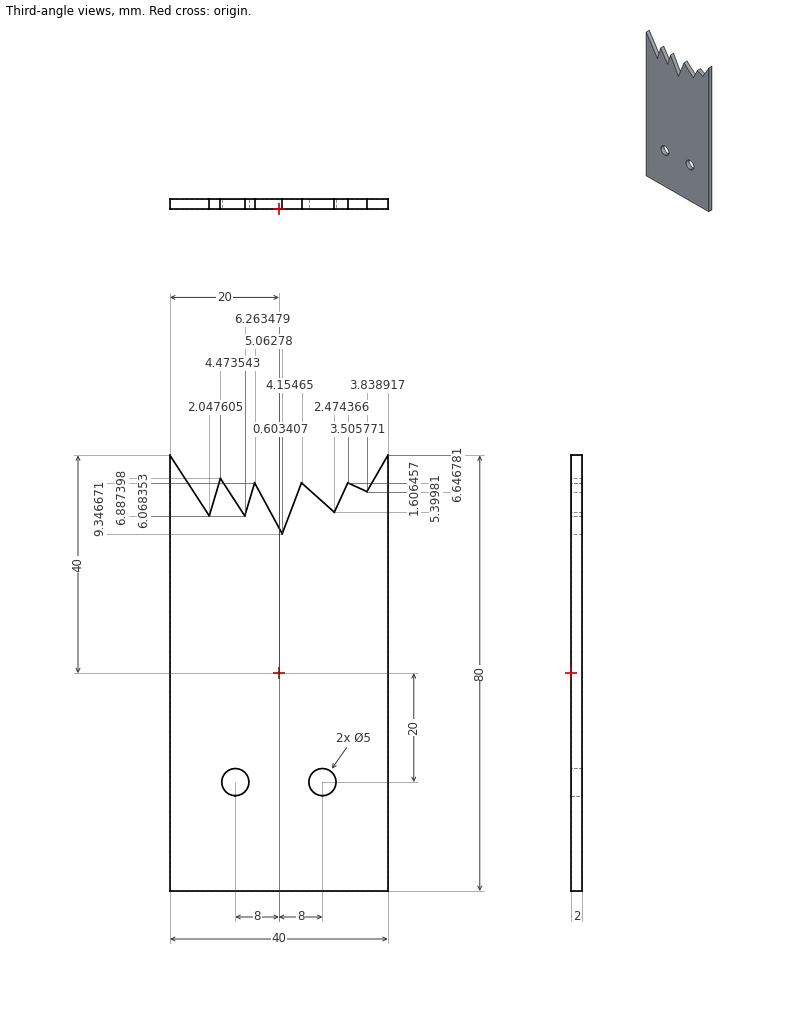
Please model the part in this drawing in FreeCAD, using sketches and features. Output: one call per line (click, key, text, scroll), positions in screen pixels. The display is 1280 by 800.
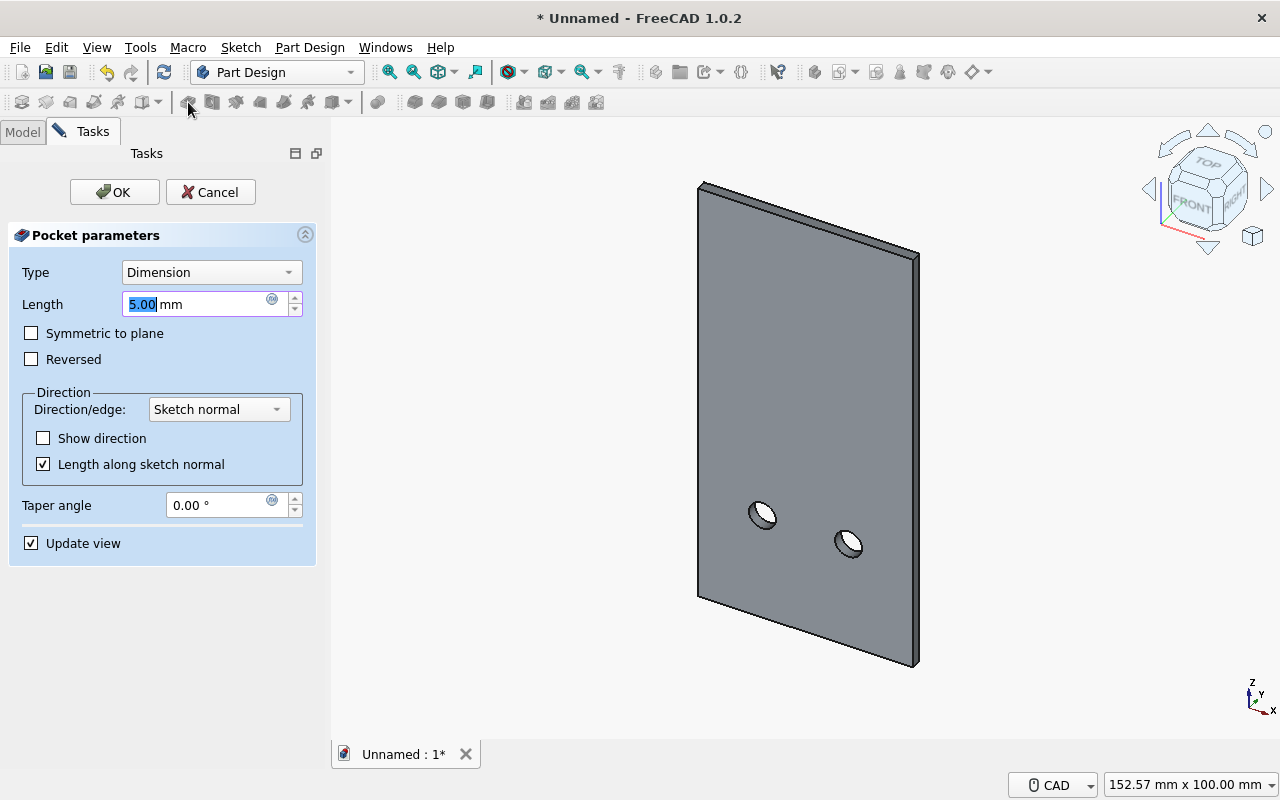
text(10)
key(Tab)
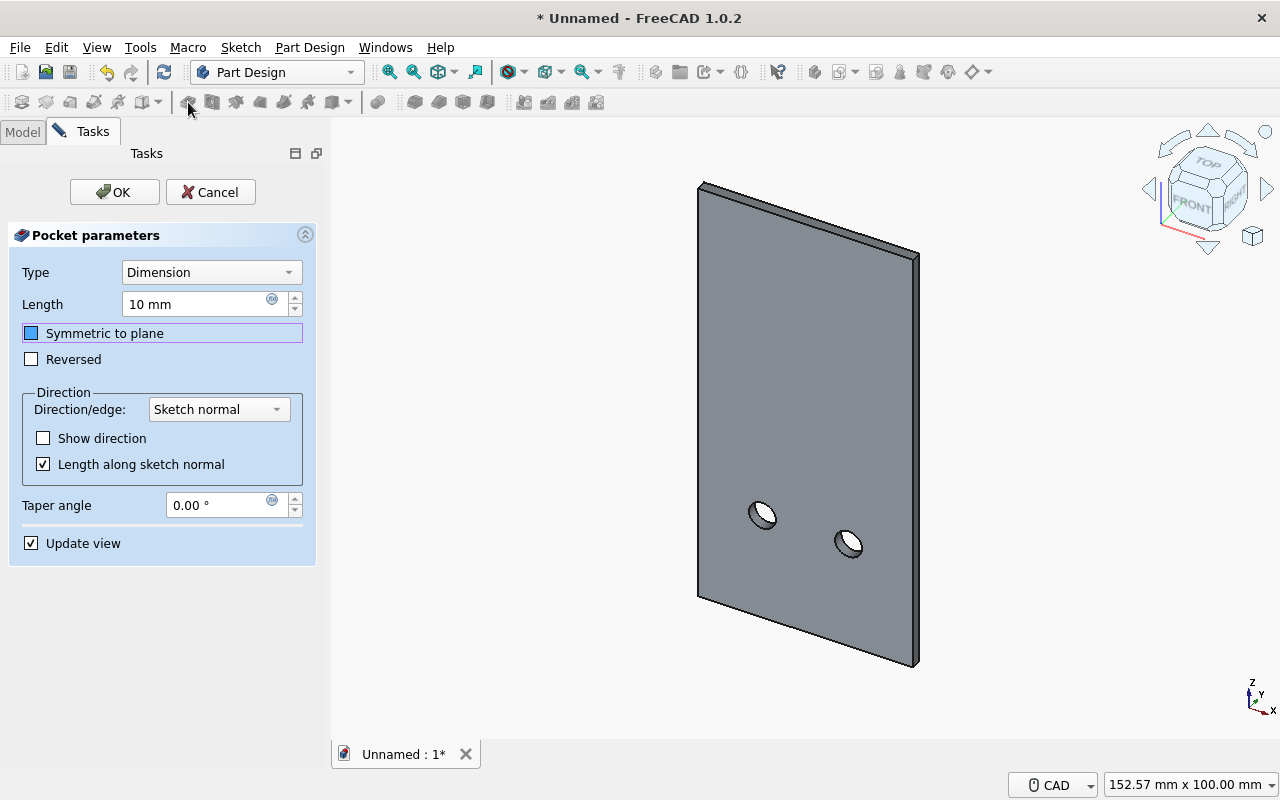
click(115, 192)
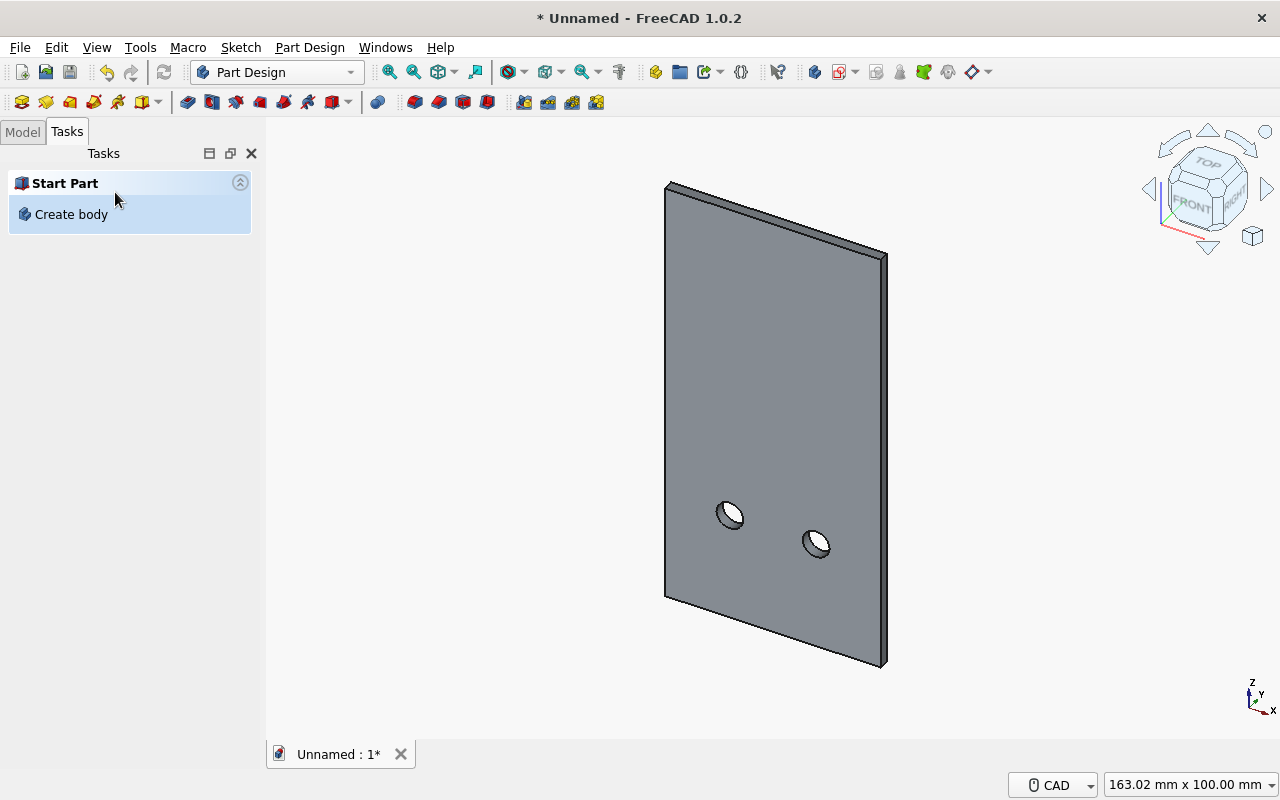
key(4)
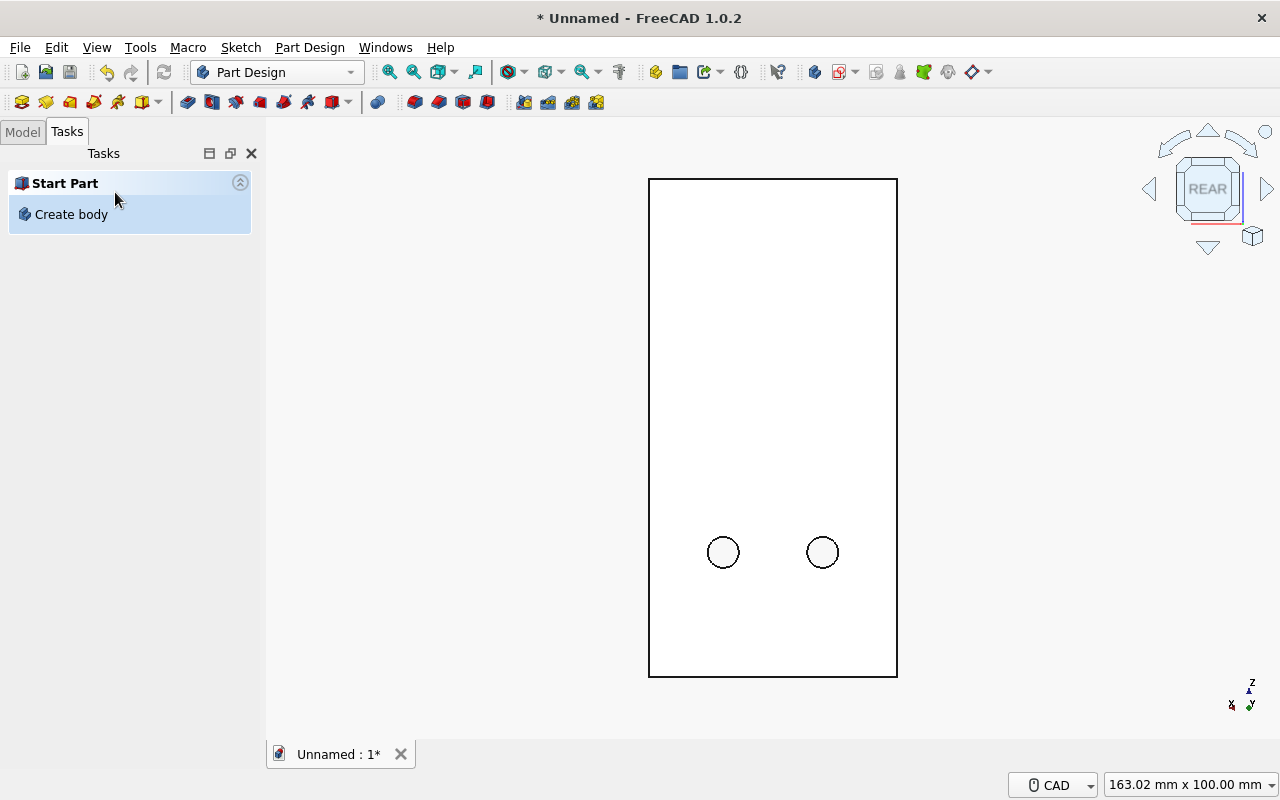
click(773, 356)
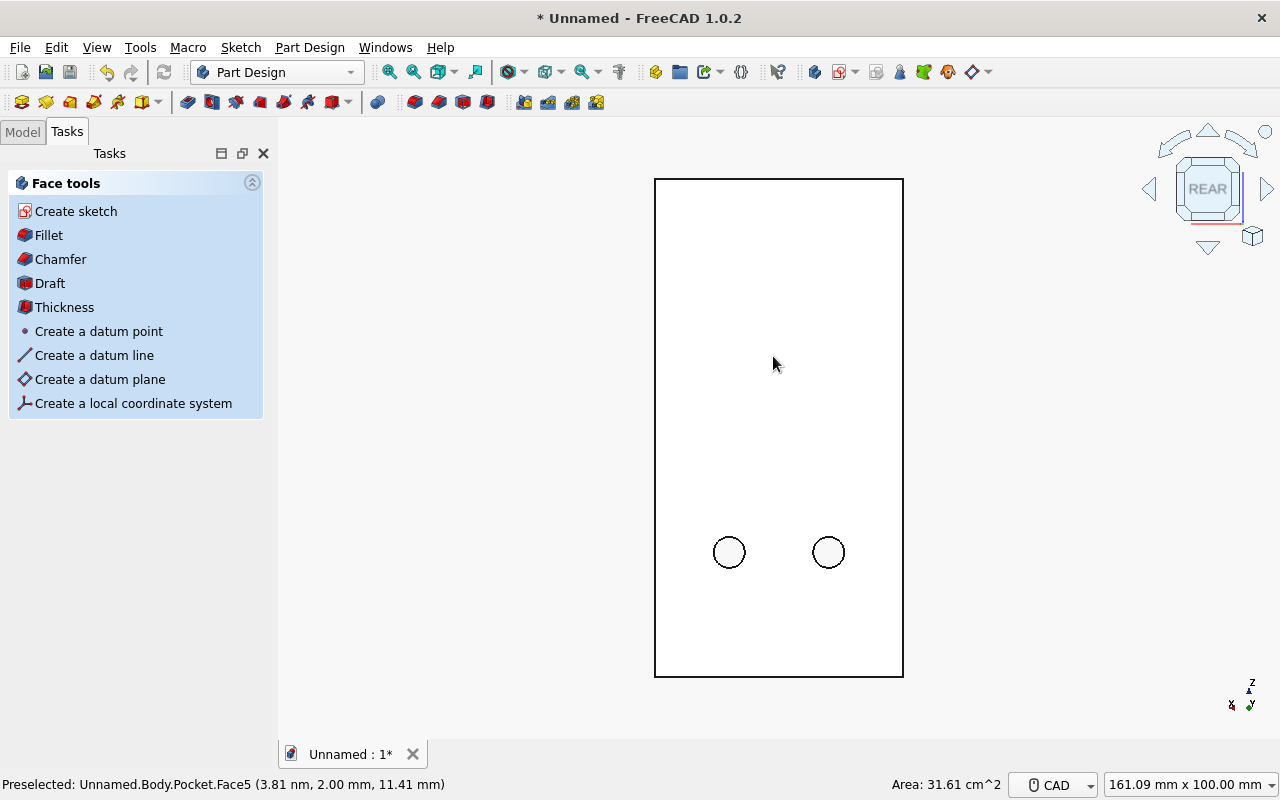
click(840, 72)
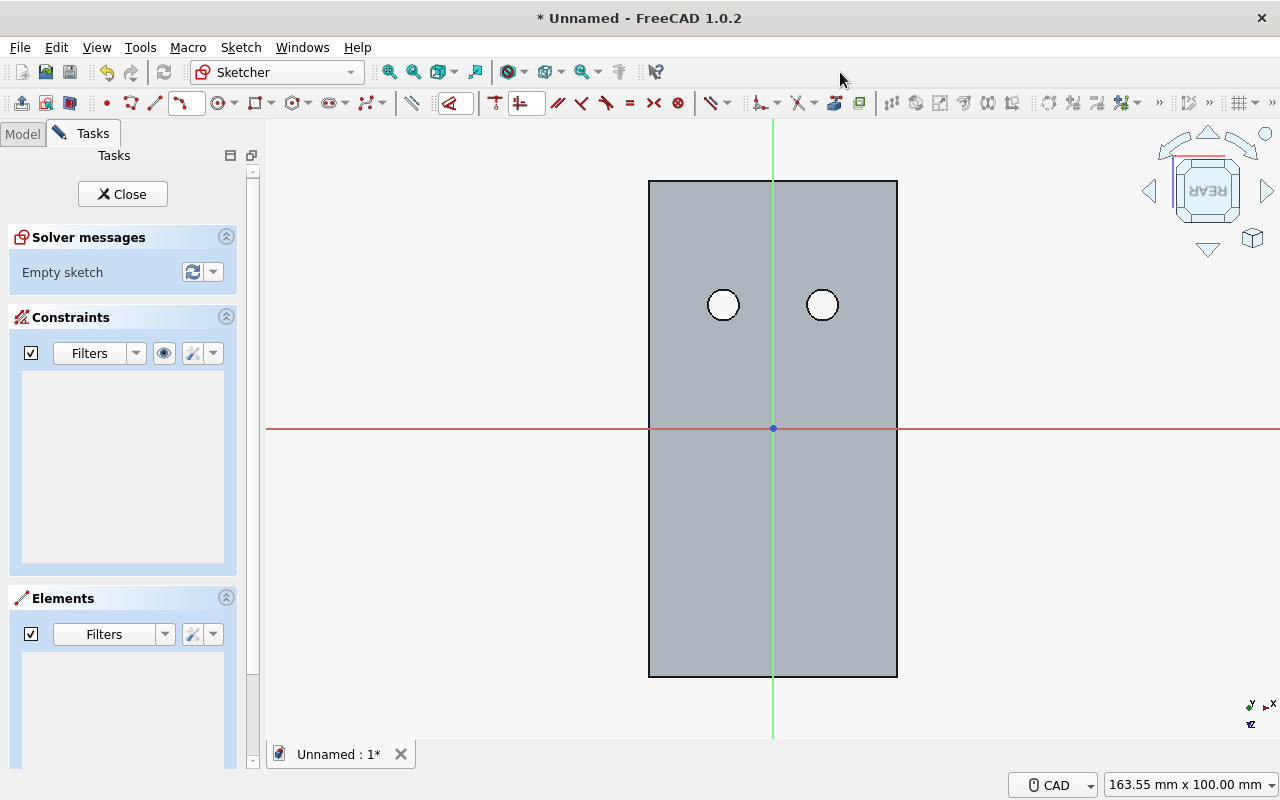
scroll(912, 711, up, 2)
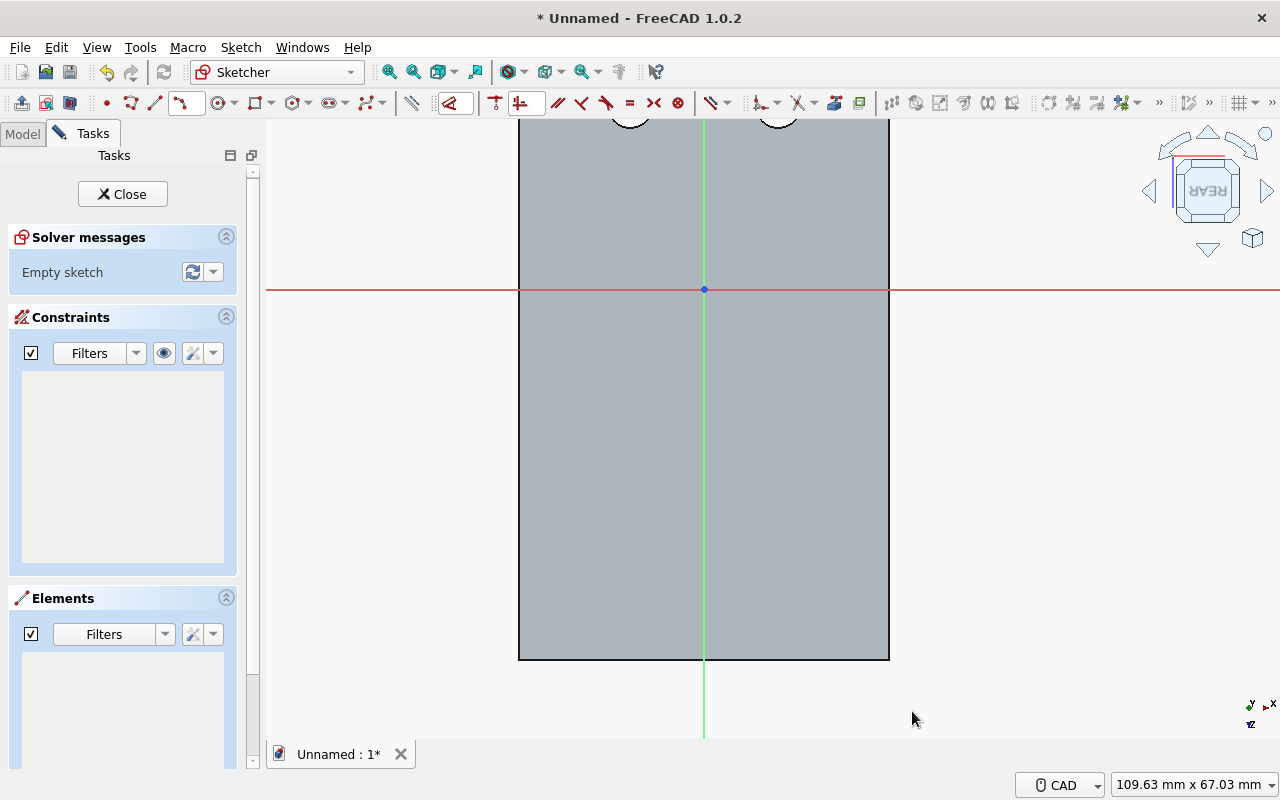
click(132, 104)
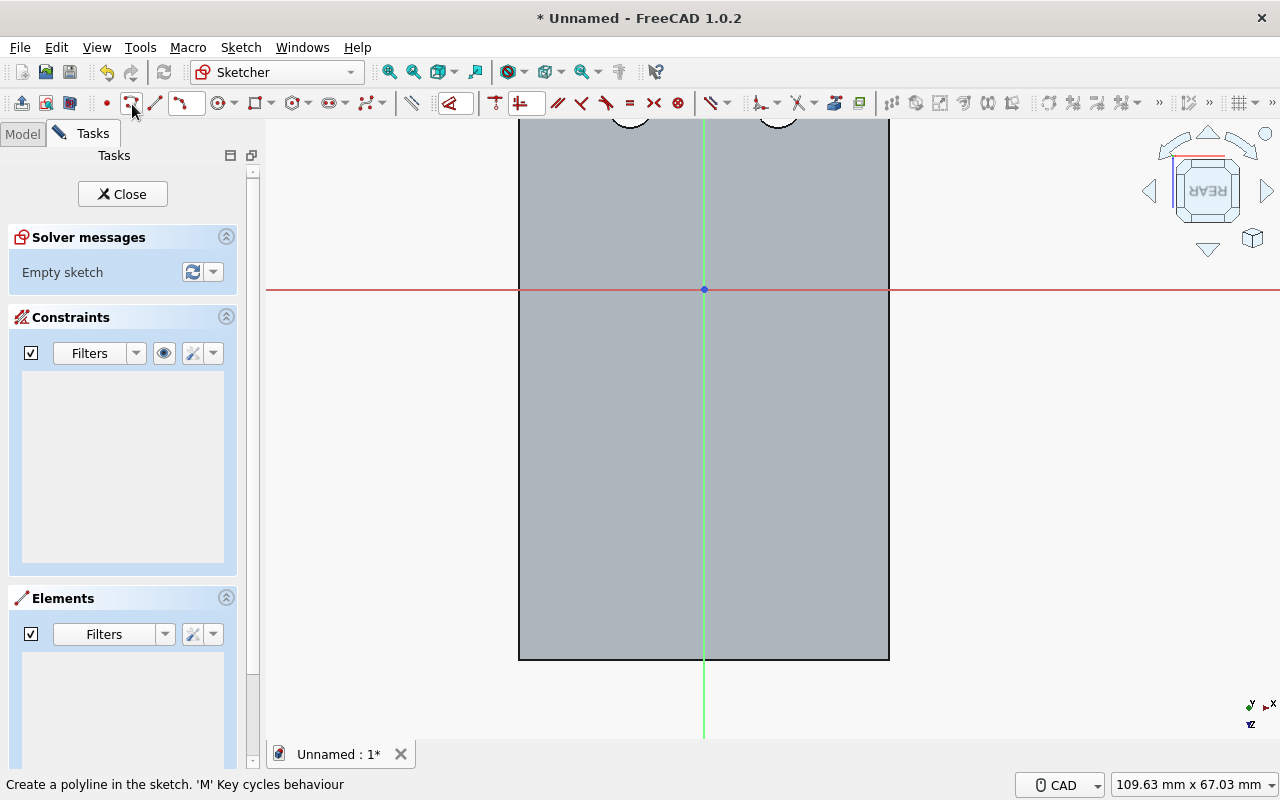
scroll(710, 527, up, 6)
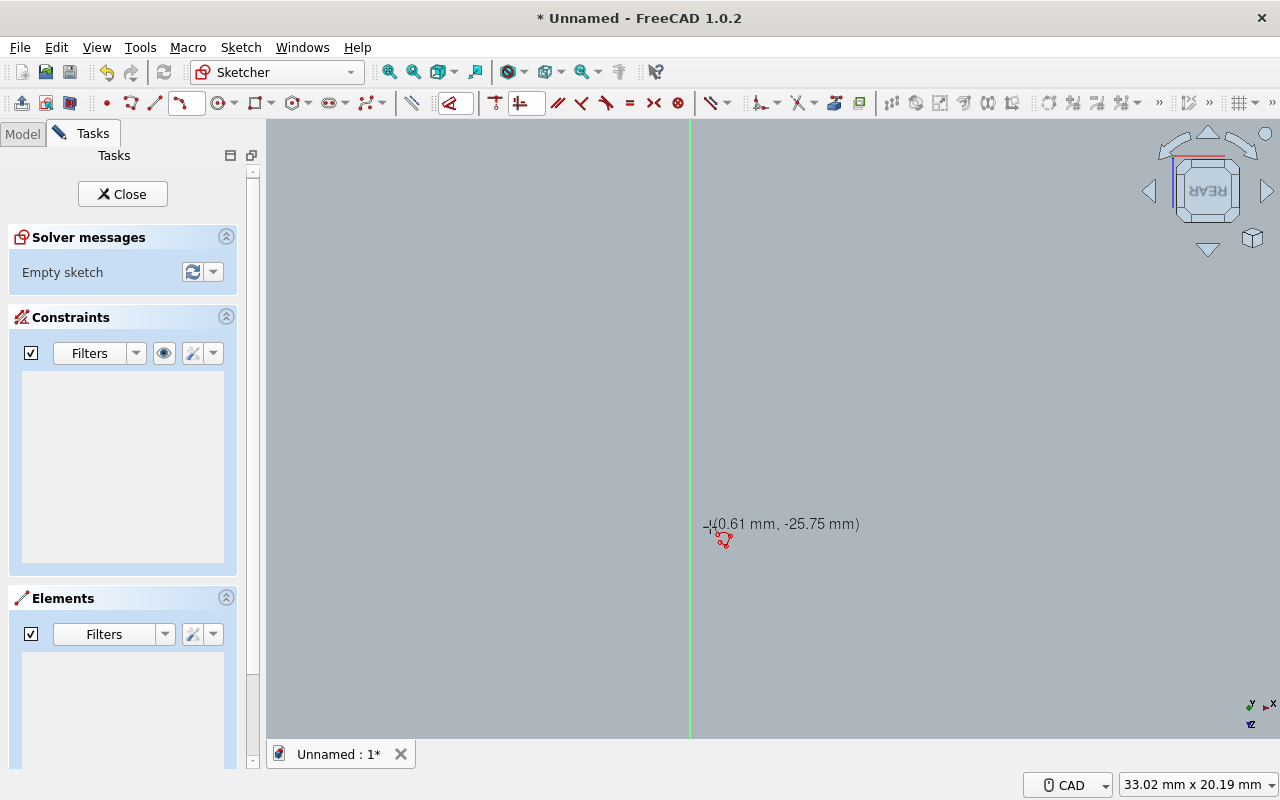
click(709, 525)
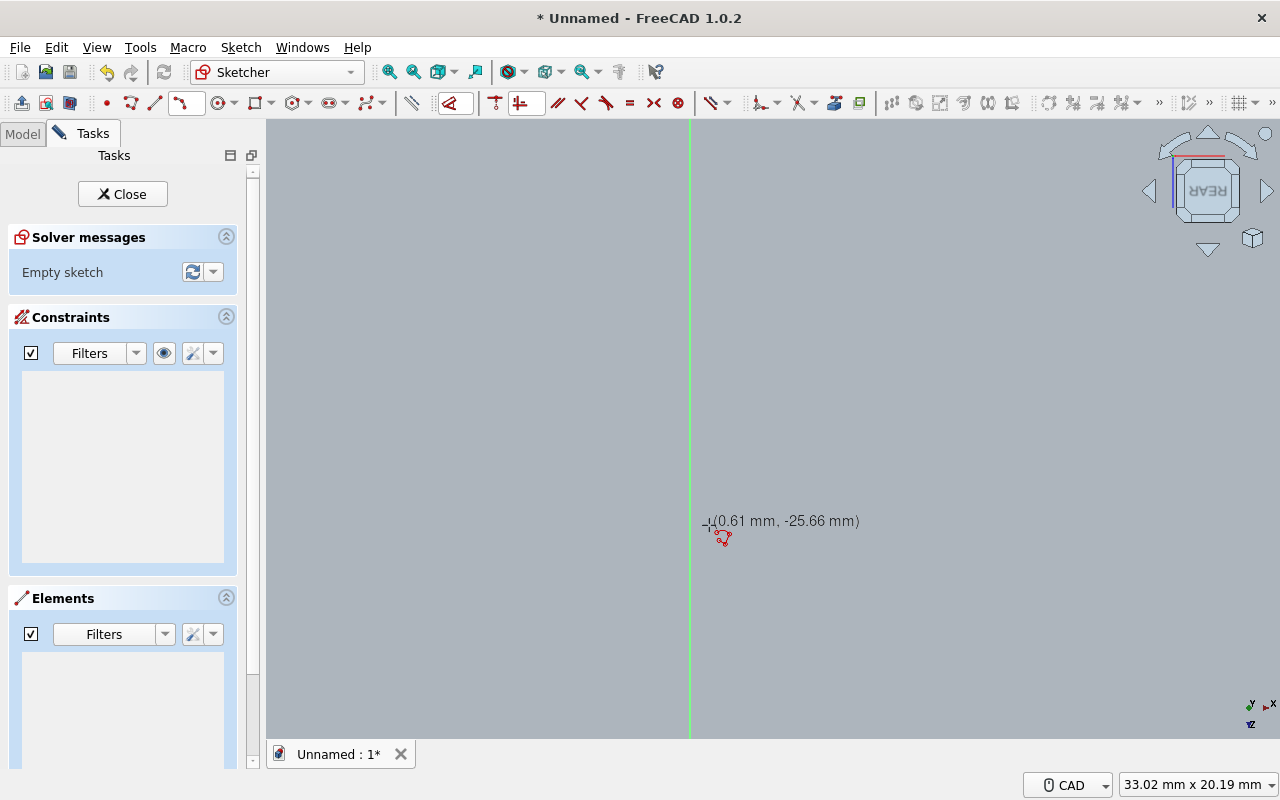
scroll(711, 462, down, 6)